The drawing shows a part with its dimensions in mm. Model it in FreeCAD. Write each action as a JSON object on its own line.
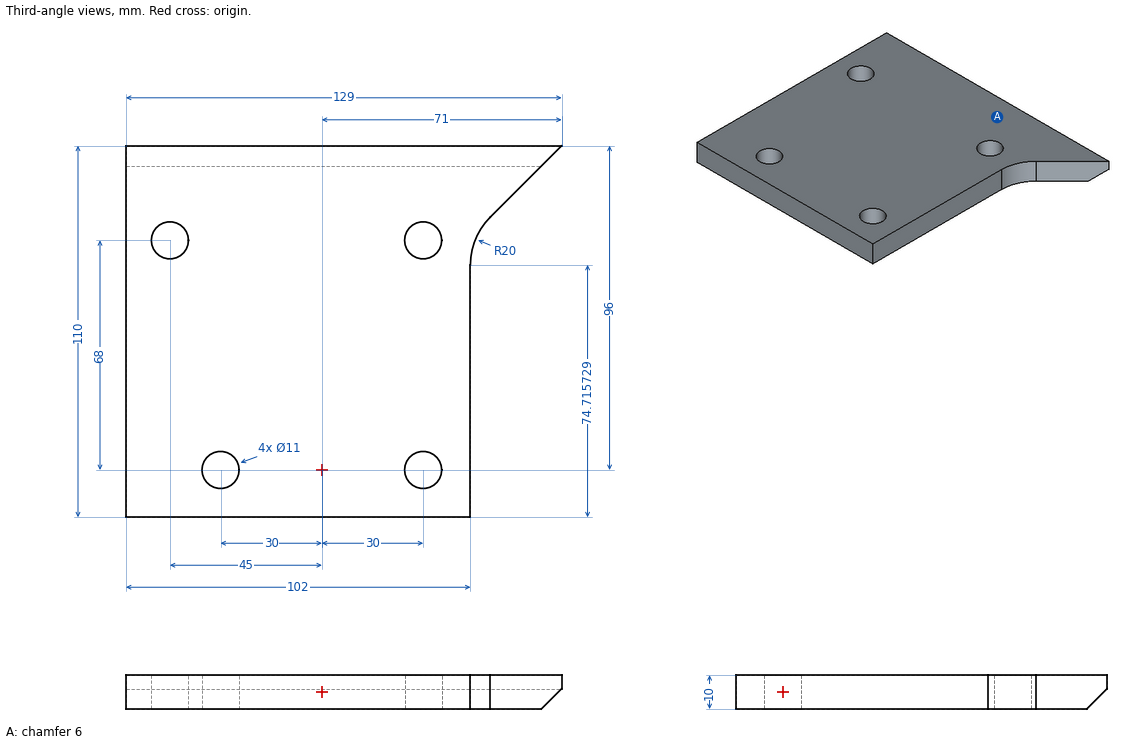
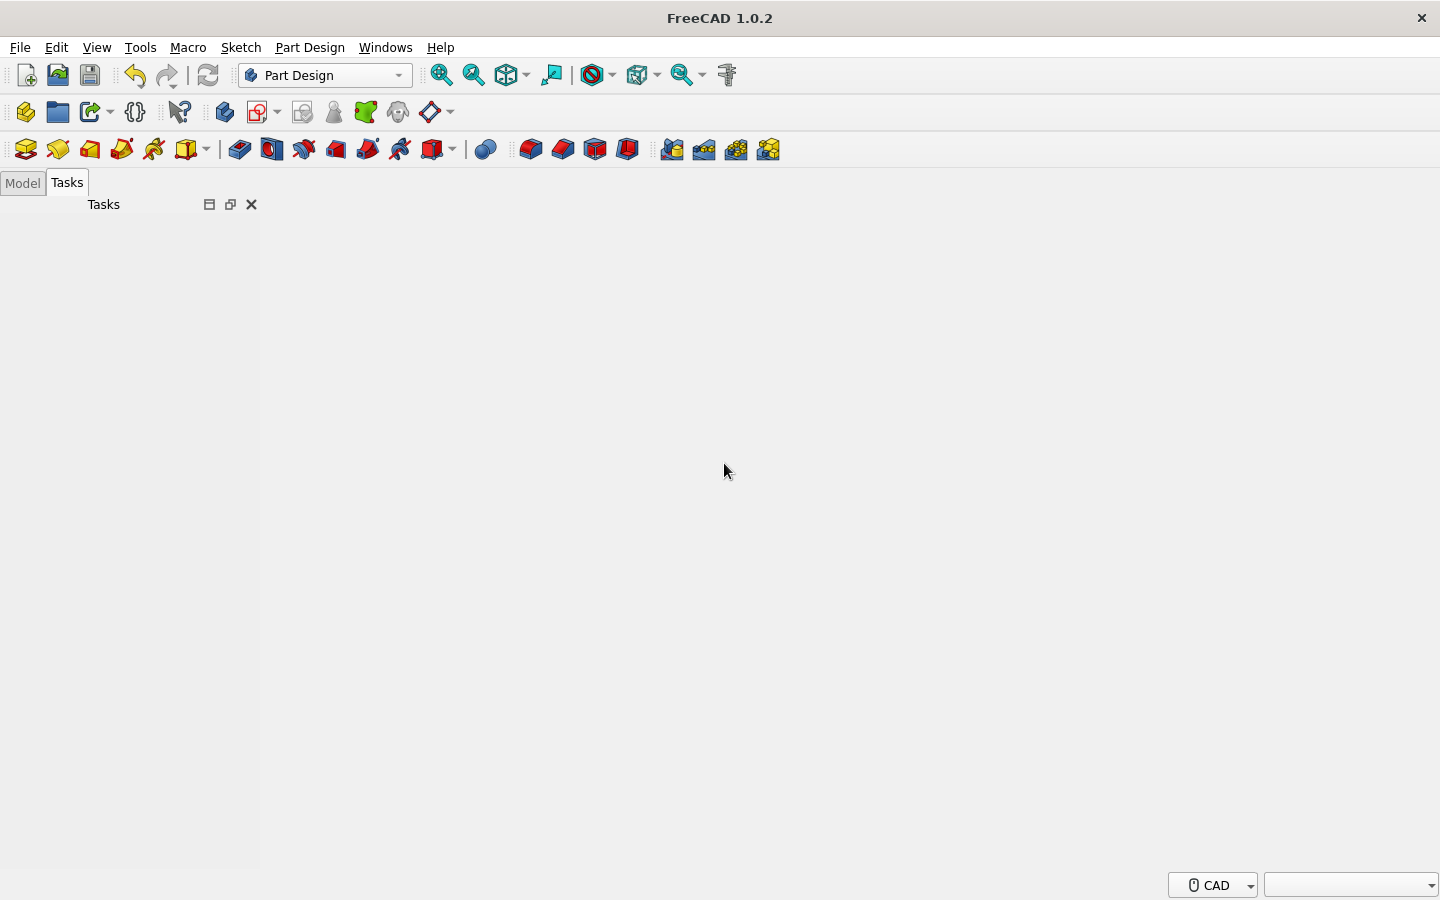
{"action": "key", "text": "ctrl+n"}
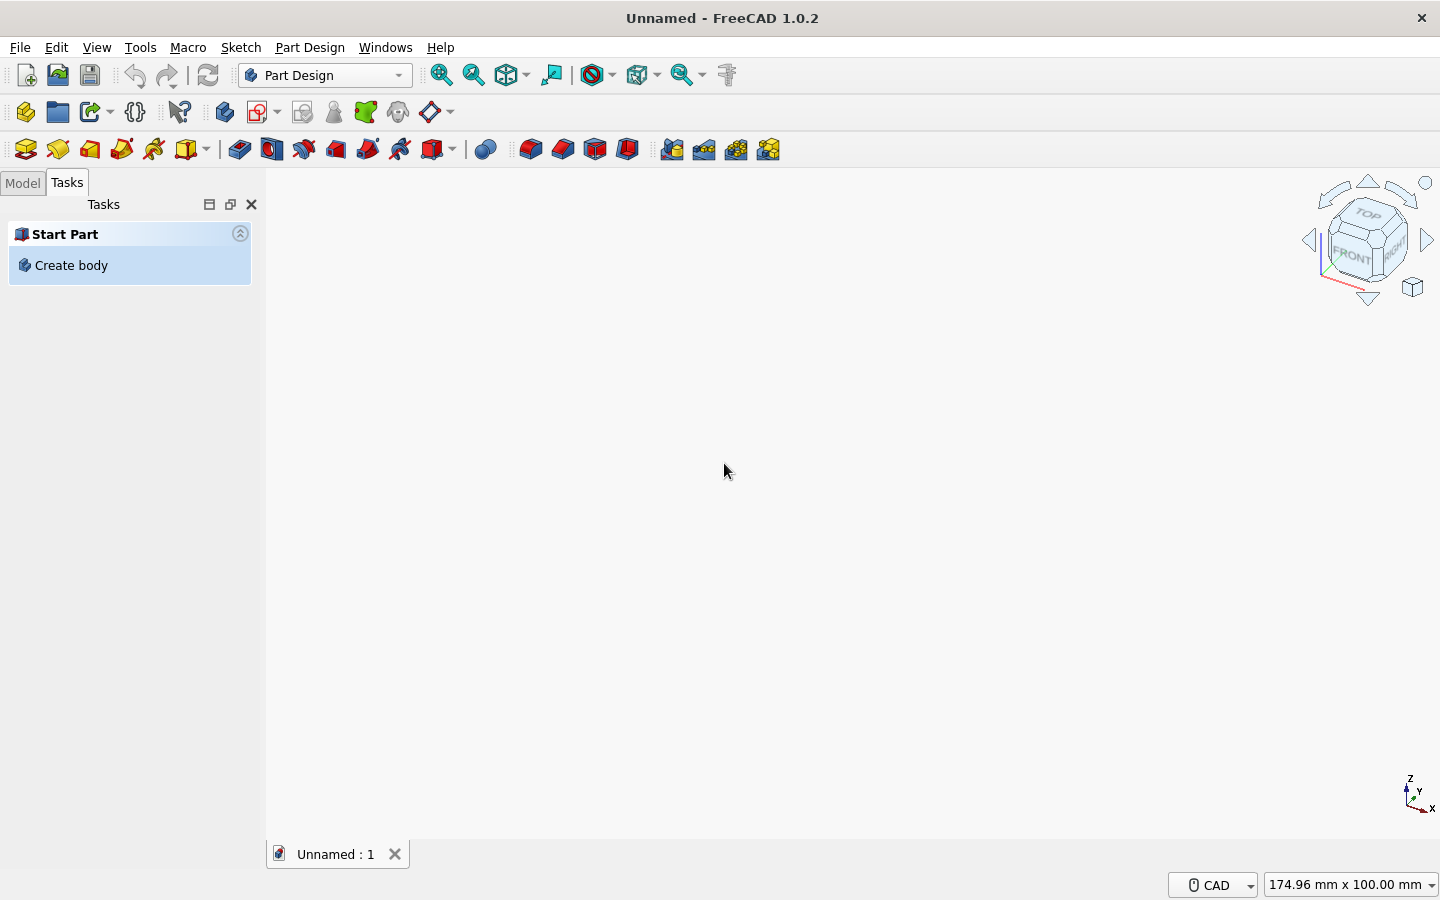
{"action": "left_click", "coordinate": [258, 112]}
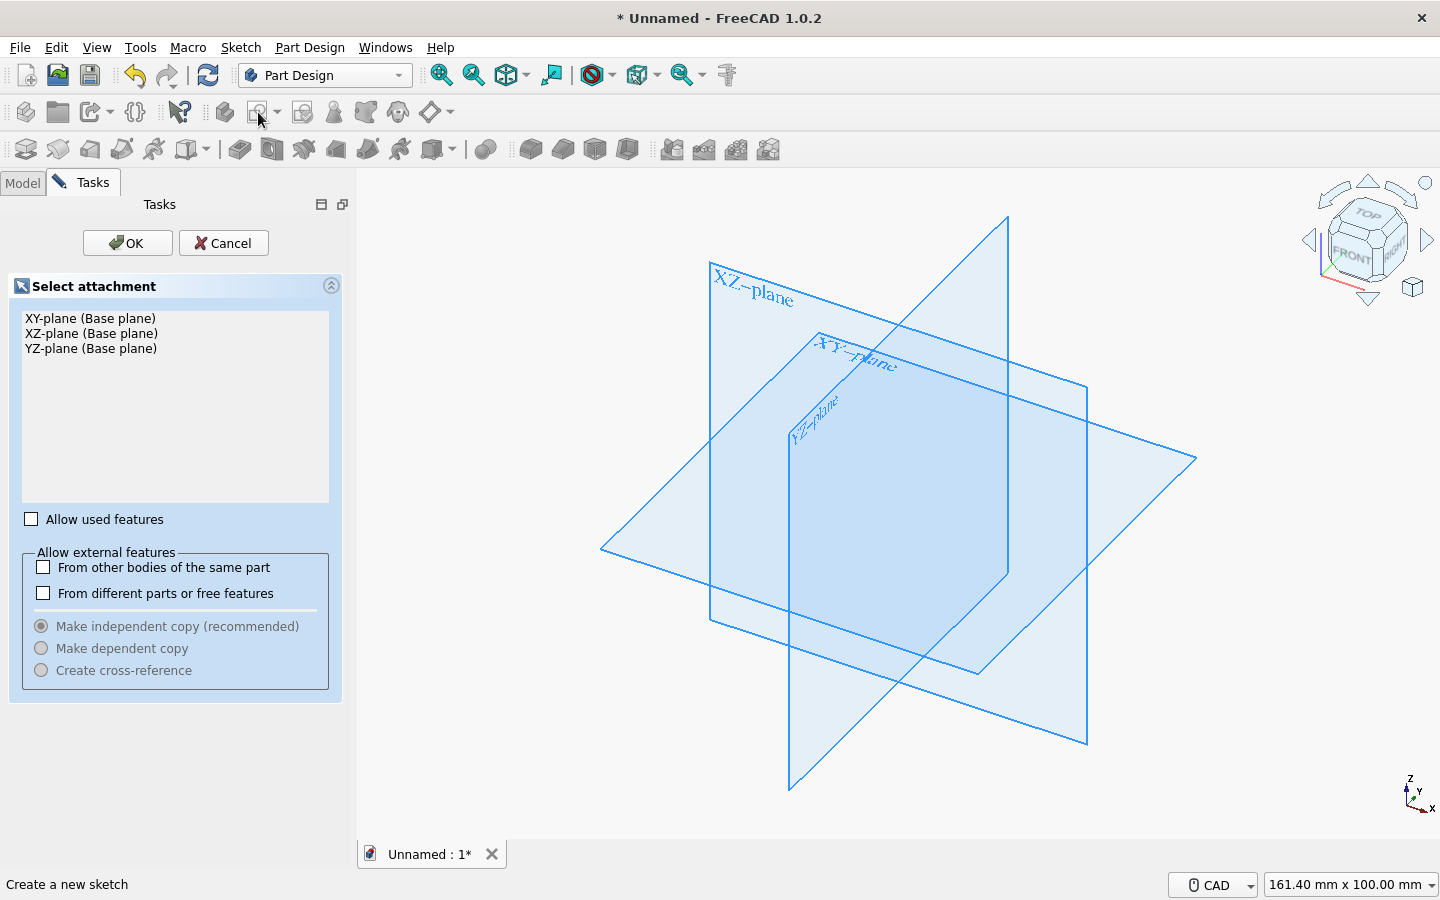
{"action": "left_click", "coordinate": [82, 318]}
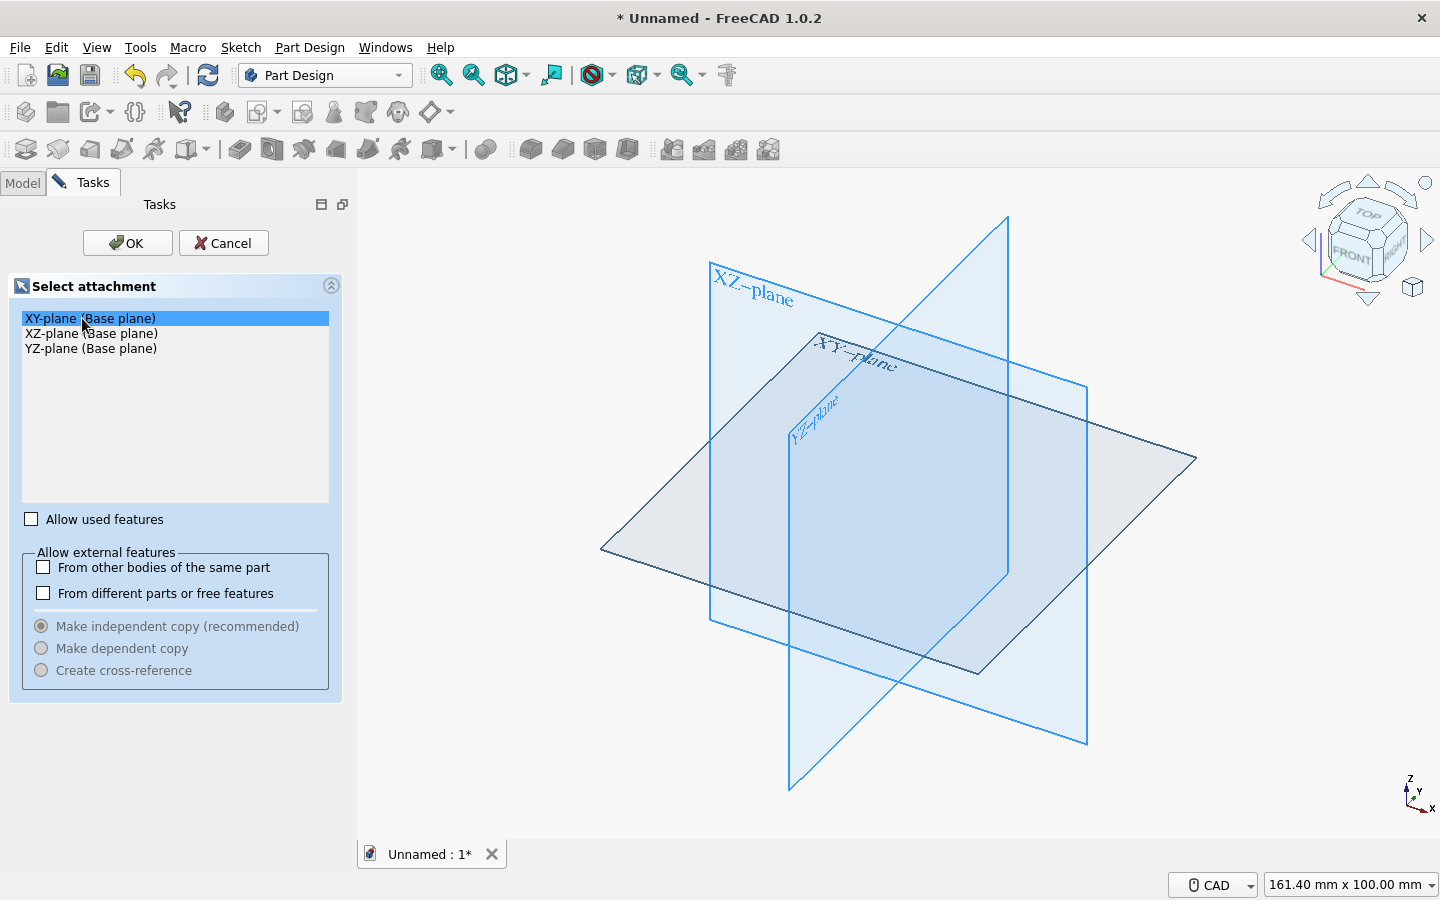
{"action": "left_click", "coordinate": [128, 243]}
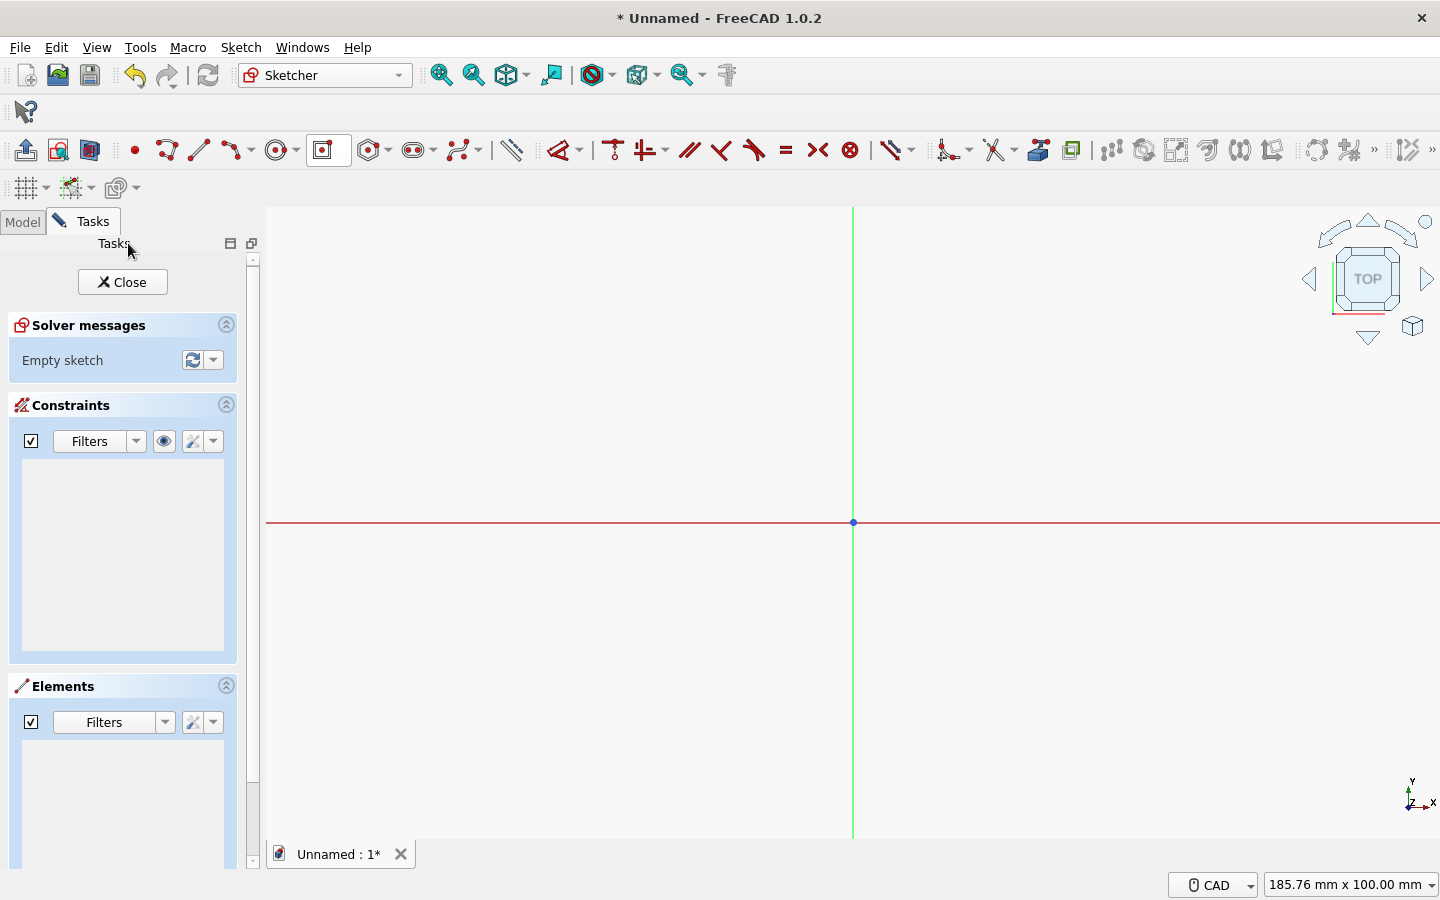
{"action": "scroll", "coordinate": [651, 811], "scroll_direction": "down", "scroll_amount": 3}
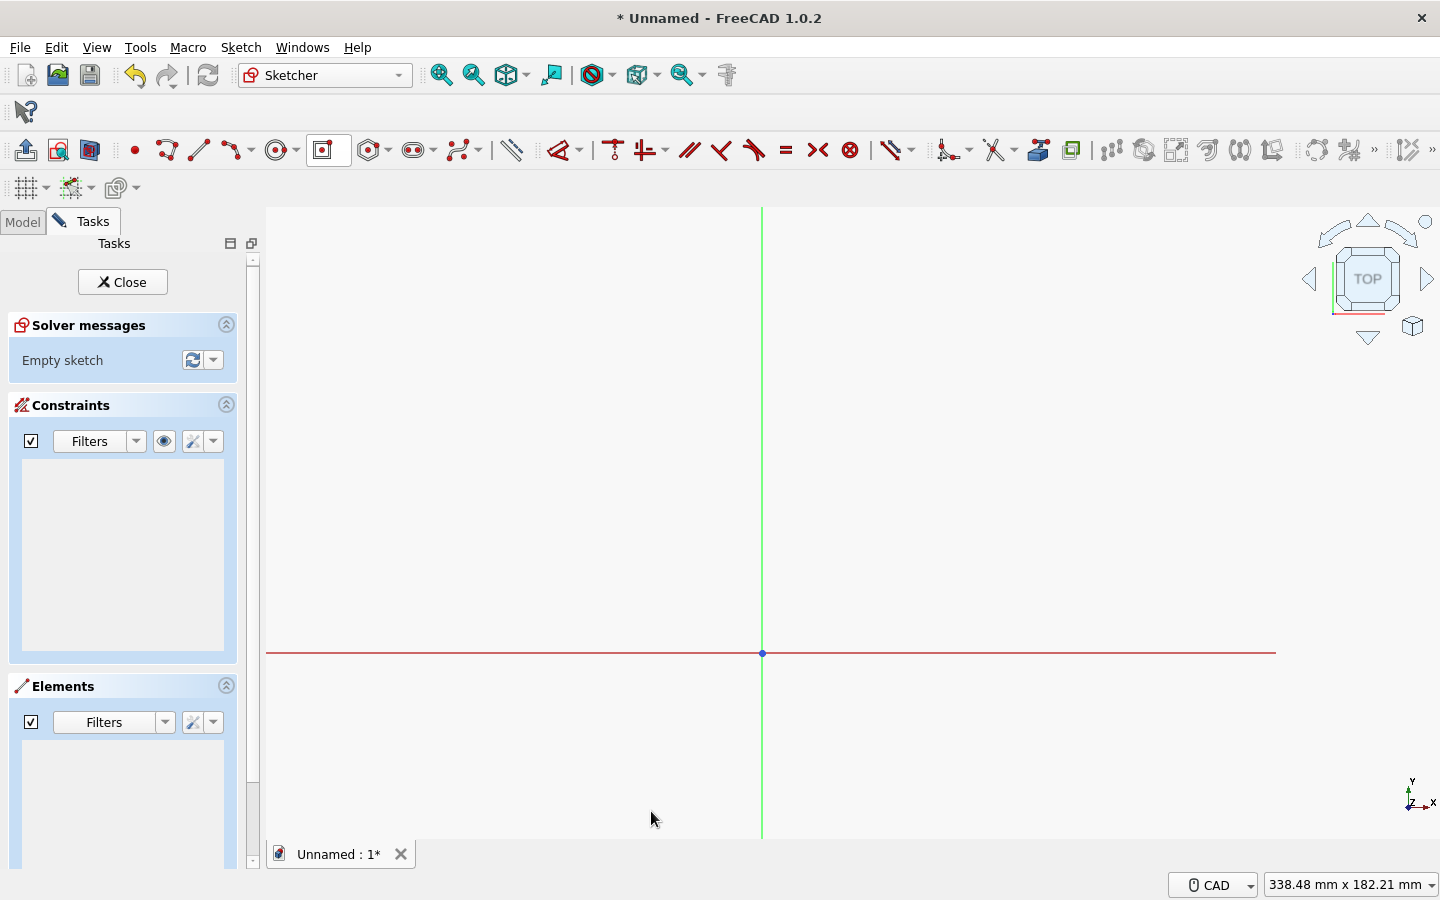
{"action": "left_click", "coordinate": [168, 150]}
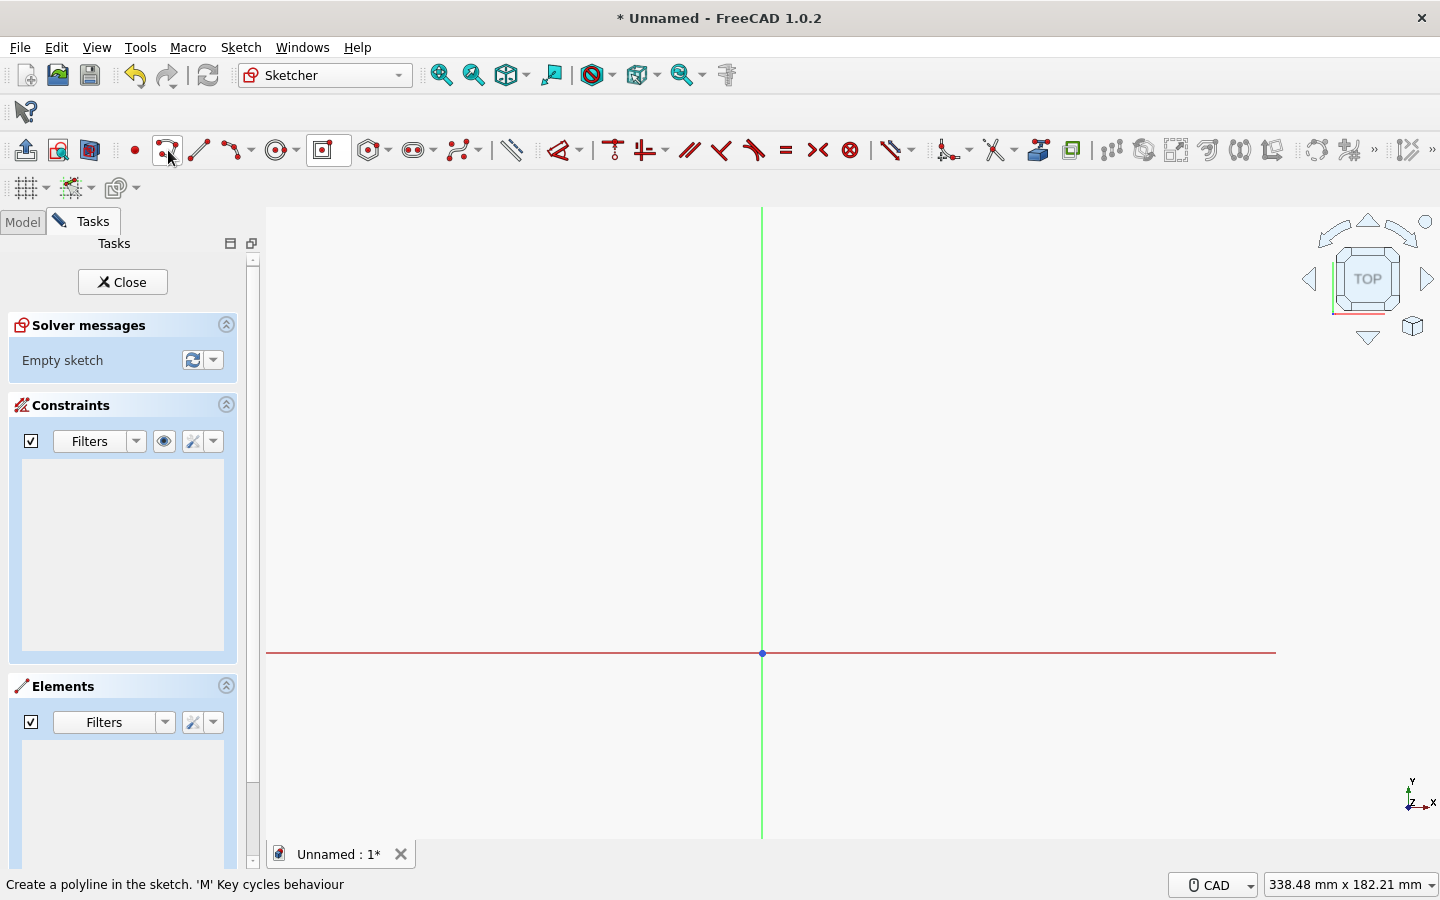
{"action": "left_click", "coordinate": [935, 394]}
{"action": "left_click", "coordinate": [1008, 320]}
{"action": "left_click", "coordinate": [561, 320]}
{"action": "left_click", "coordinate": [561, 702]}
{"action": "left_click", "coordinate": [915, 702]}
{"action": "left_click", "coordinate": [915, 443]}
{"action": "right_click", "coordinate": [915, 443]}